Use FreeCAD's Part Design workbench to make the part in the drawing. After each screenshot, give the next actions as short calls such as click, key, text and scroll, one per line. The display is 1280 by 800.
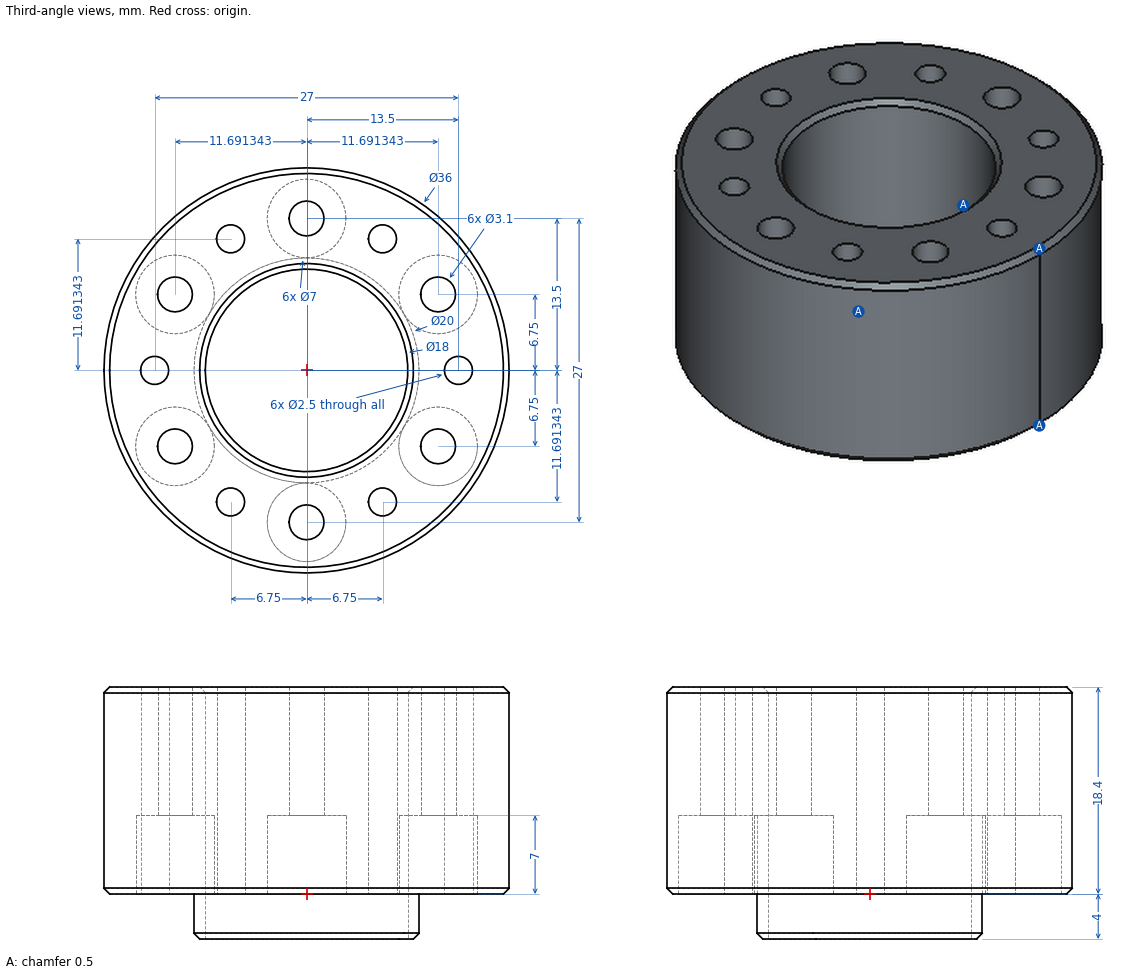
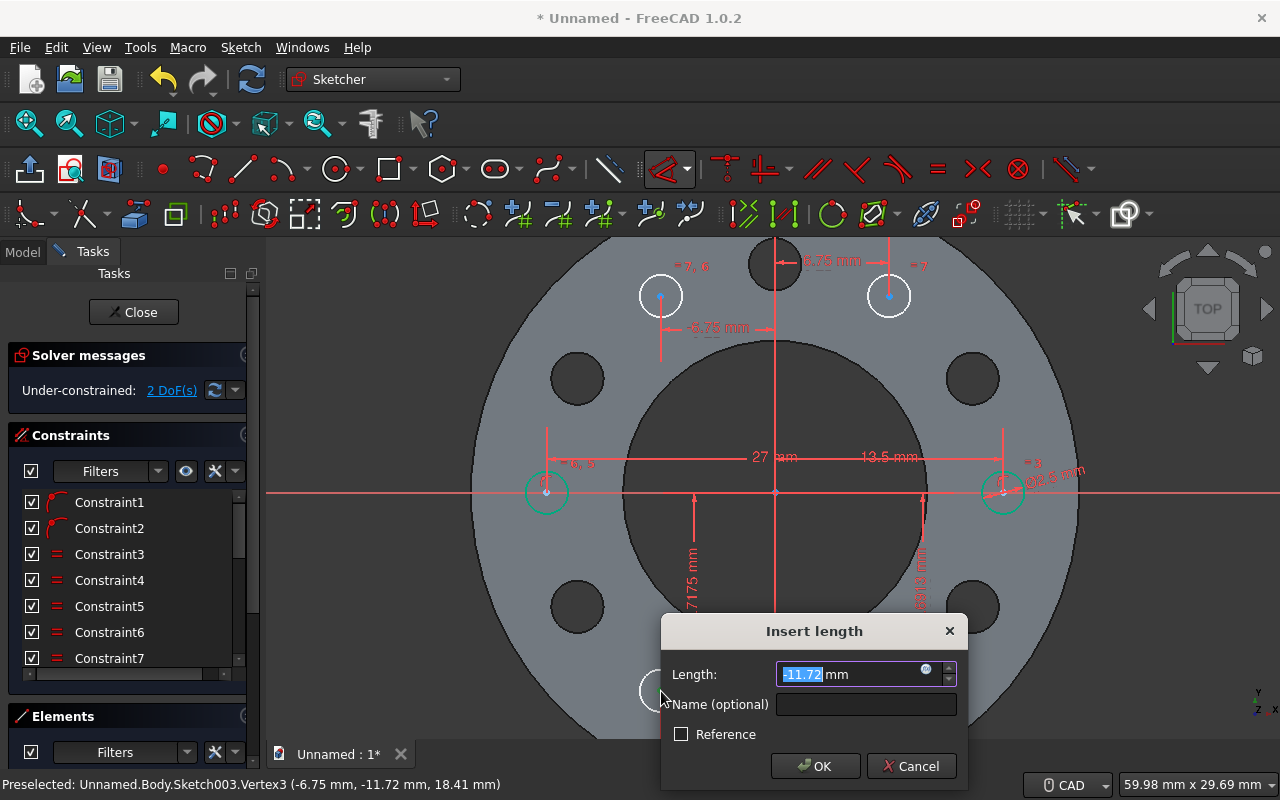
text(-11.691343)
key(Return)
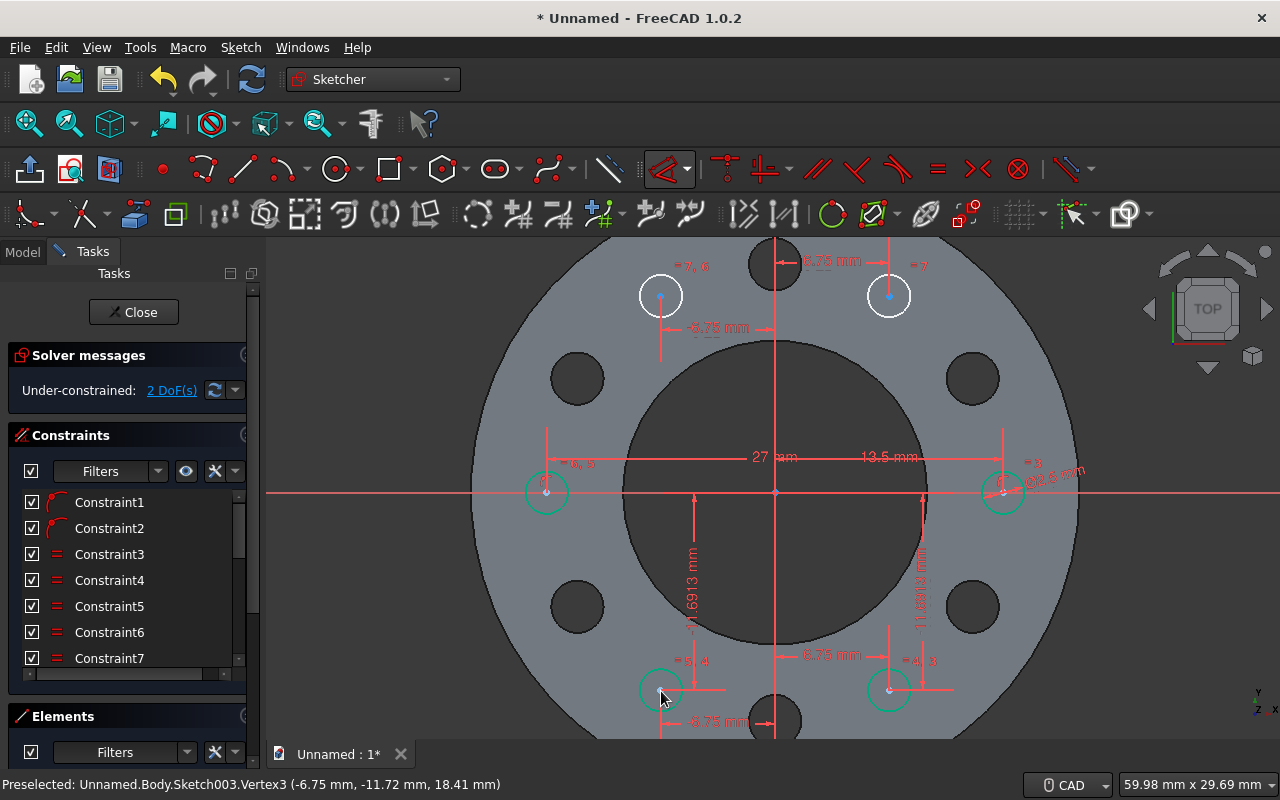
click(661, 296)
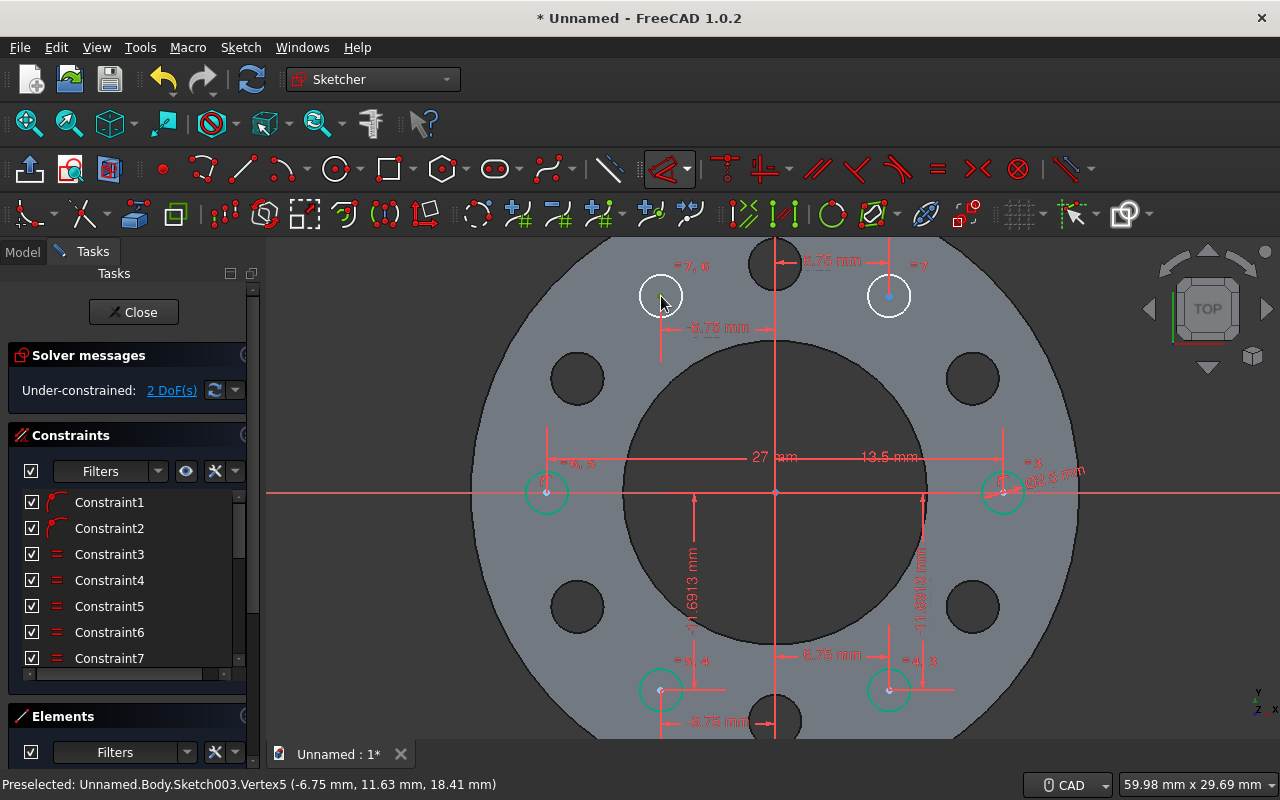
key(i)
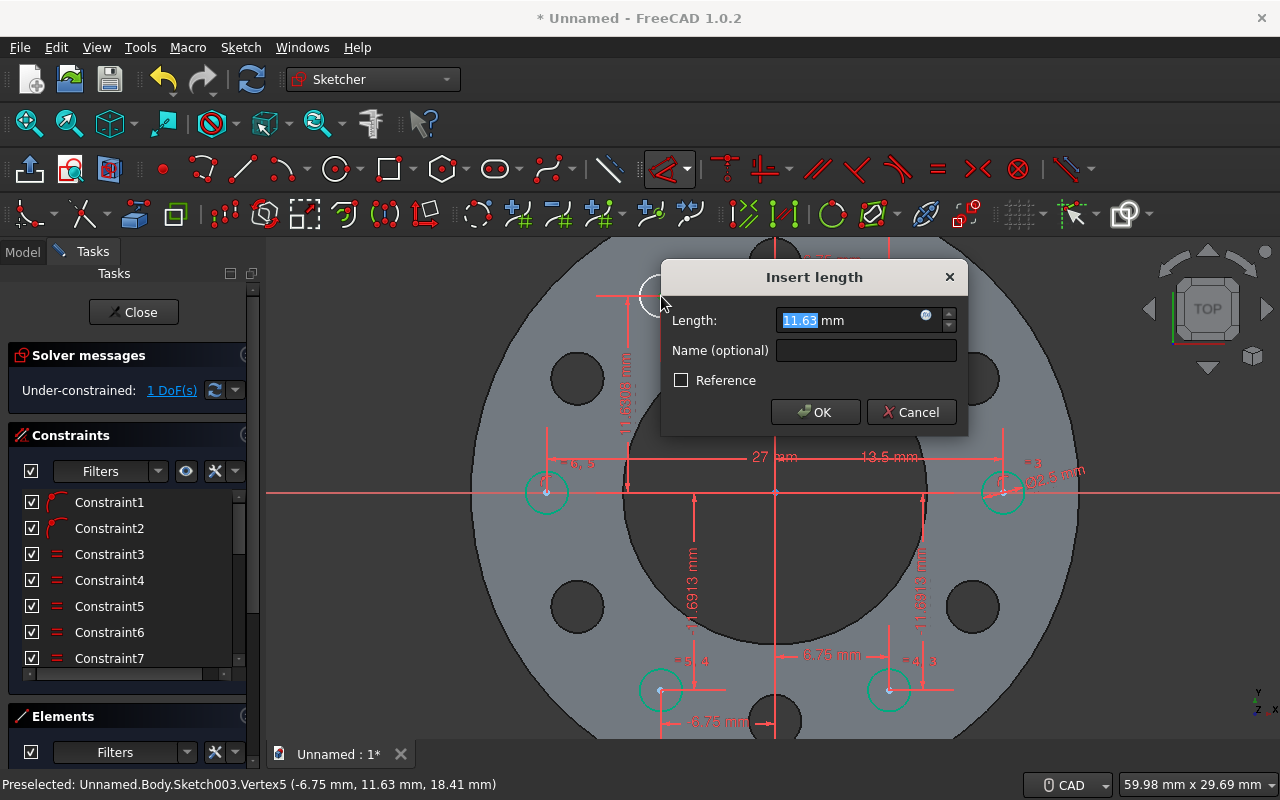
text(11.691343)
key(Return)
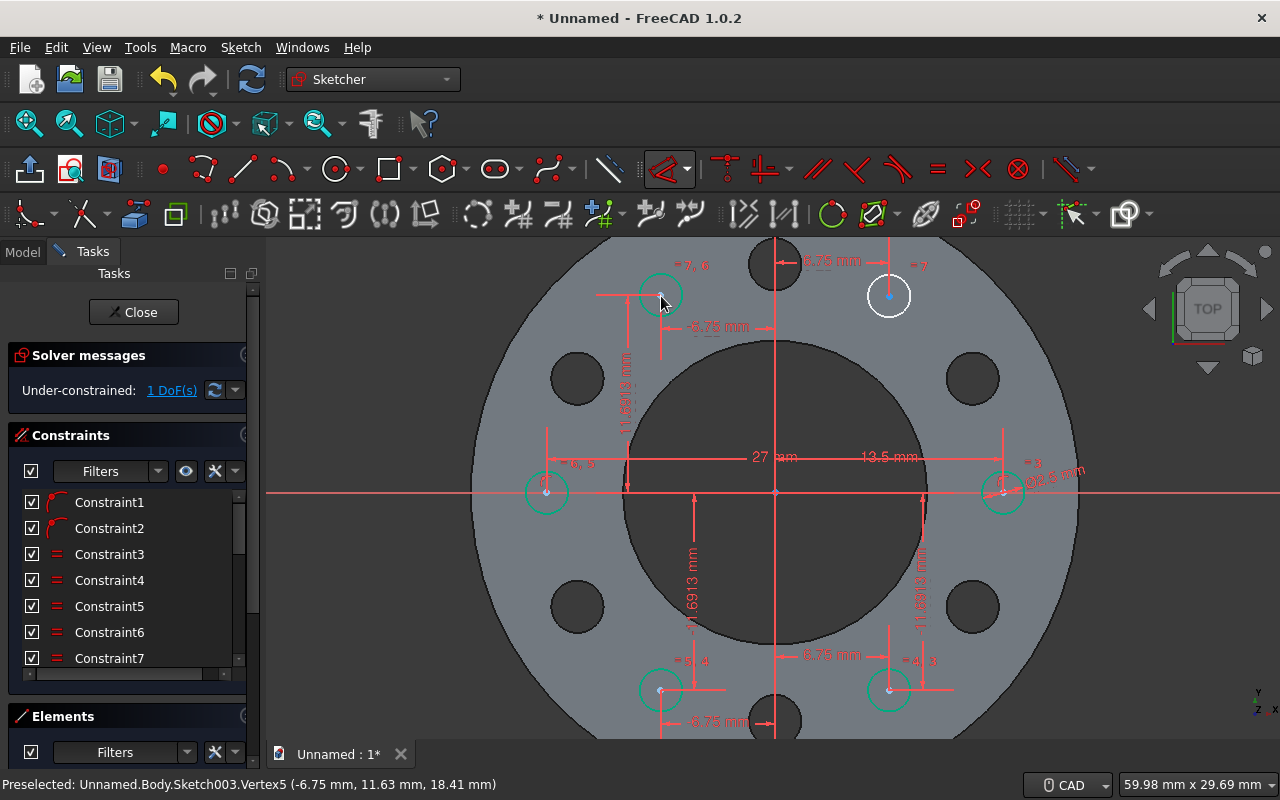
click(889, 296)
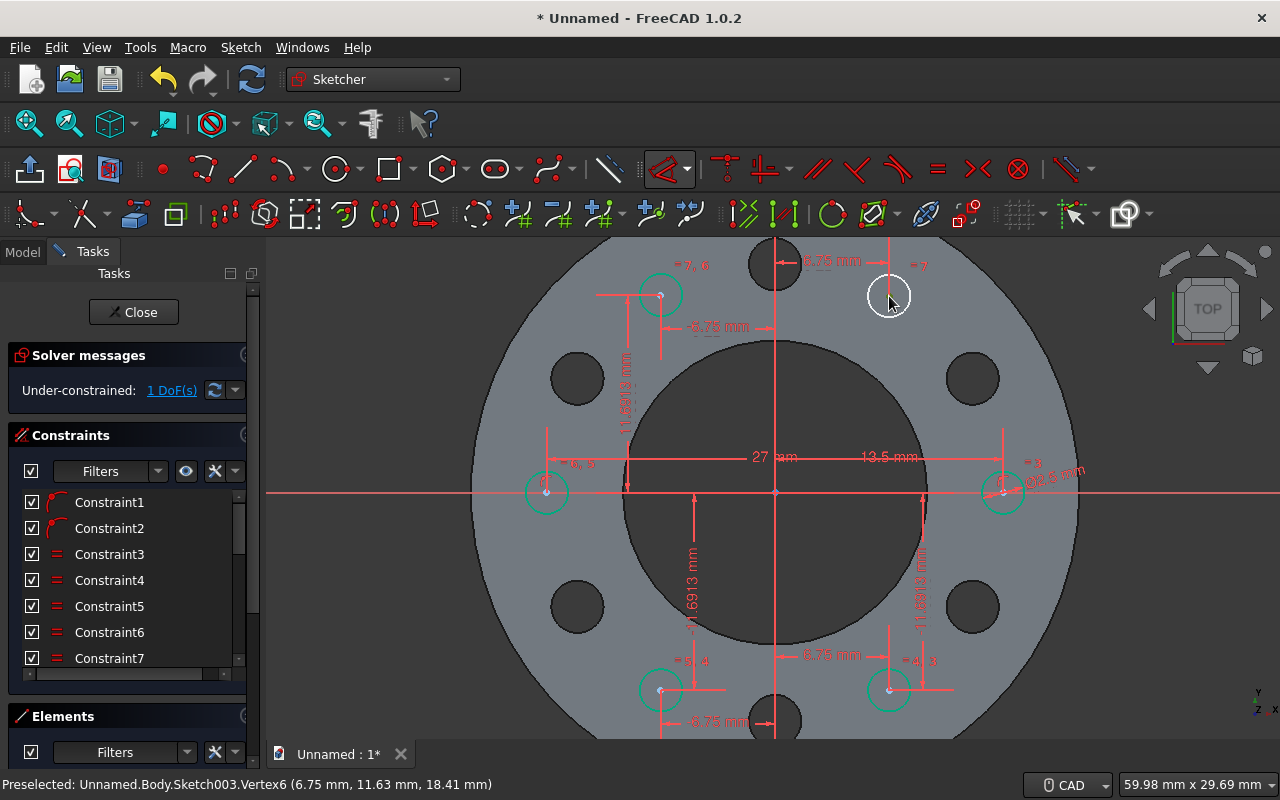
key(i)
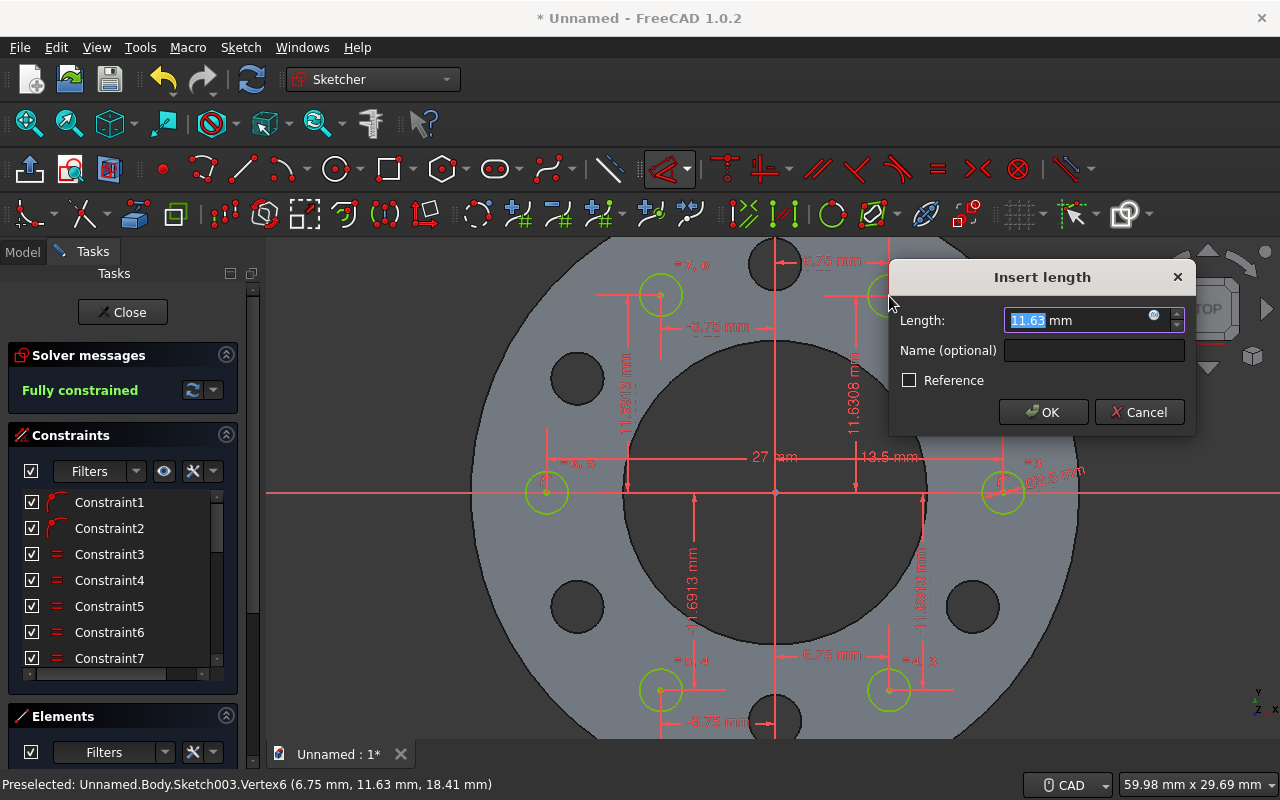
text(11.691343)
key(Return)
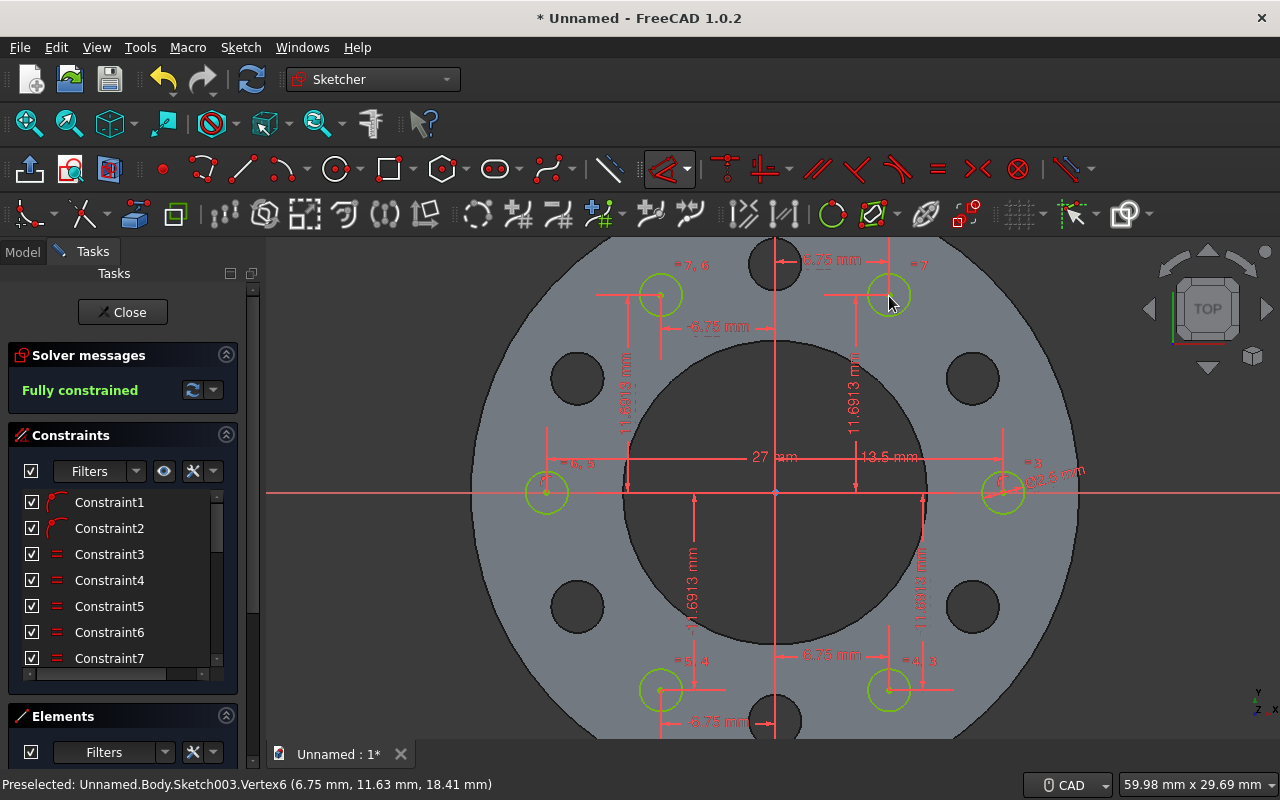
click(123, 312)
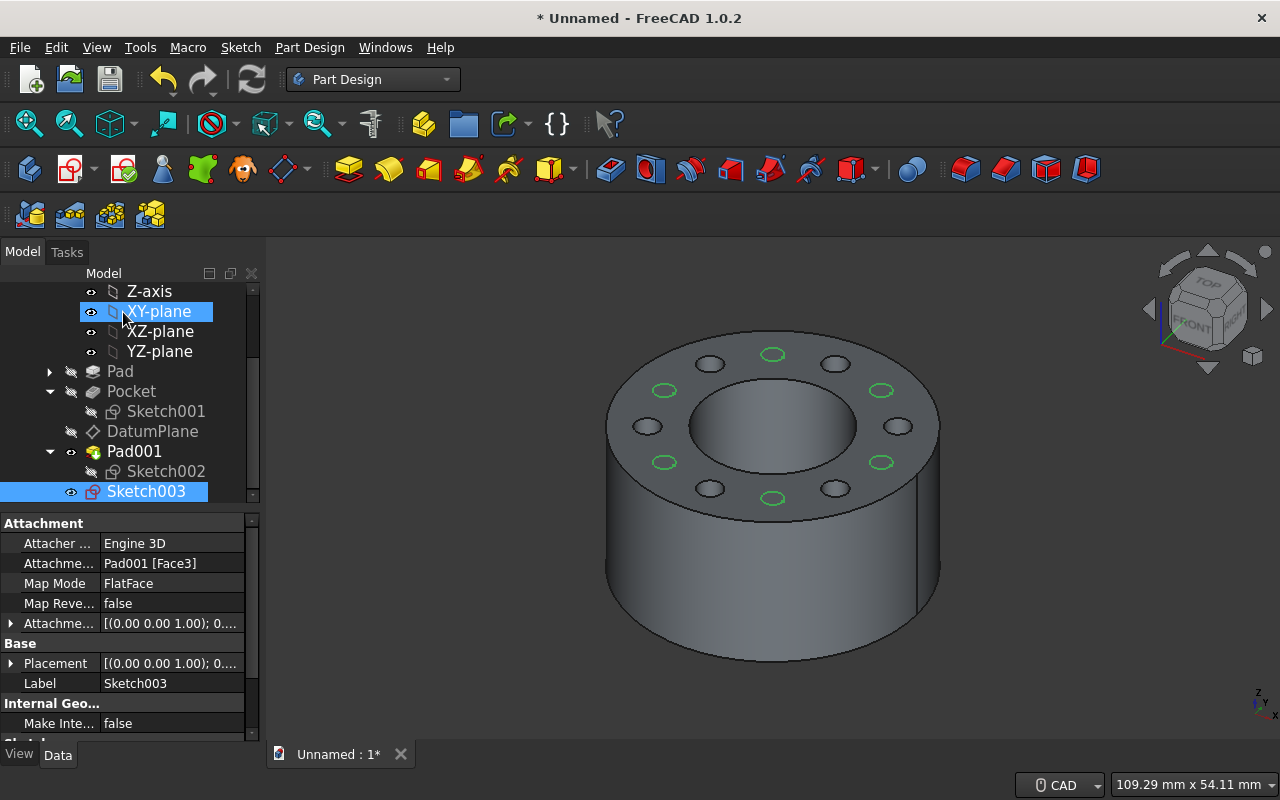
click(652, 170)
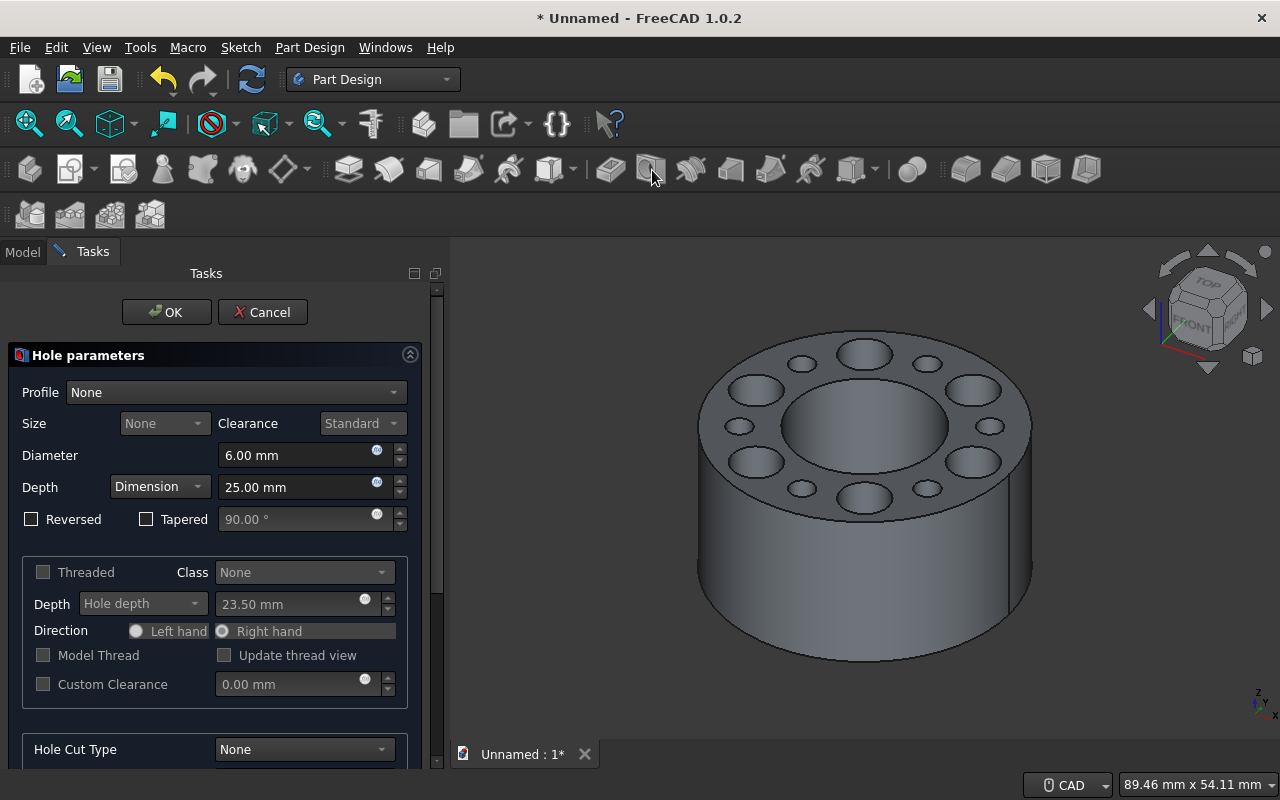
triple_click(305, 455)